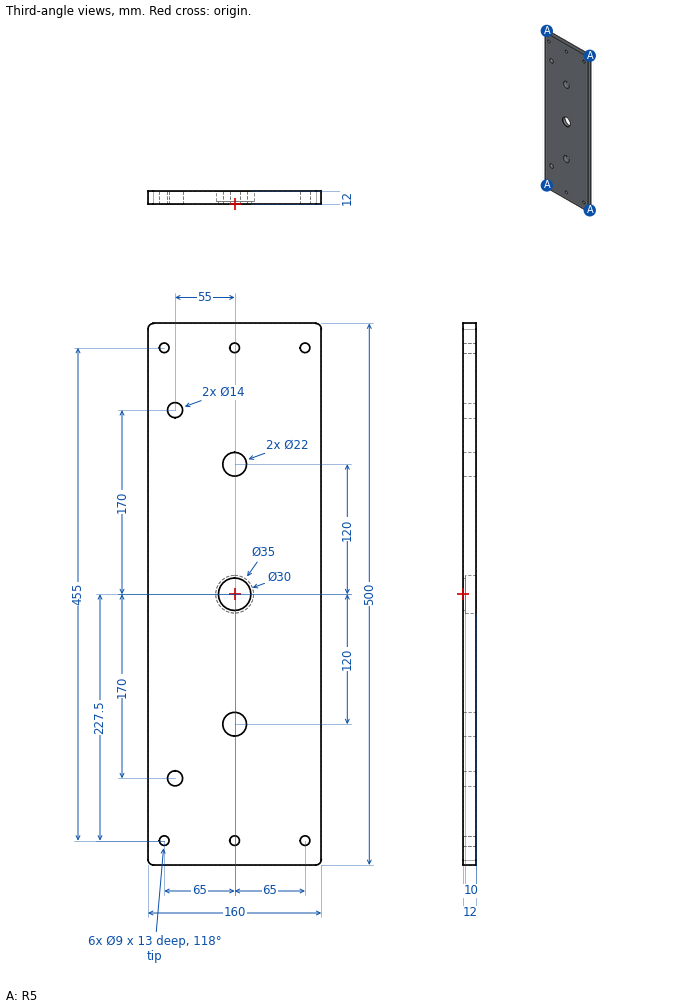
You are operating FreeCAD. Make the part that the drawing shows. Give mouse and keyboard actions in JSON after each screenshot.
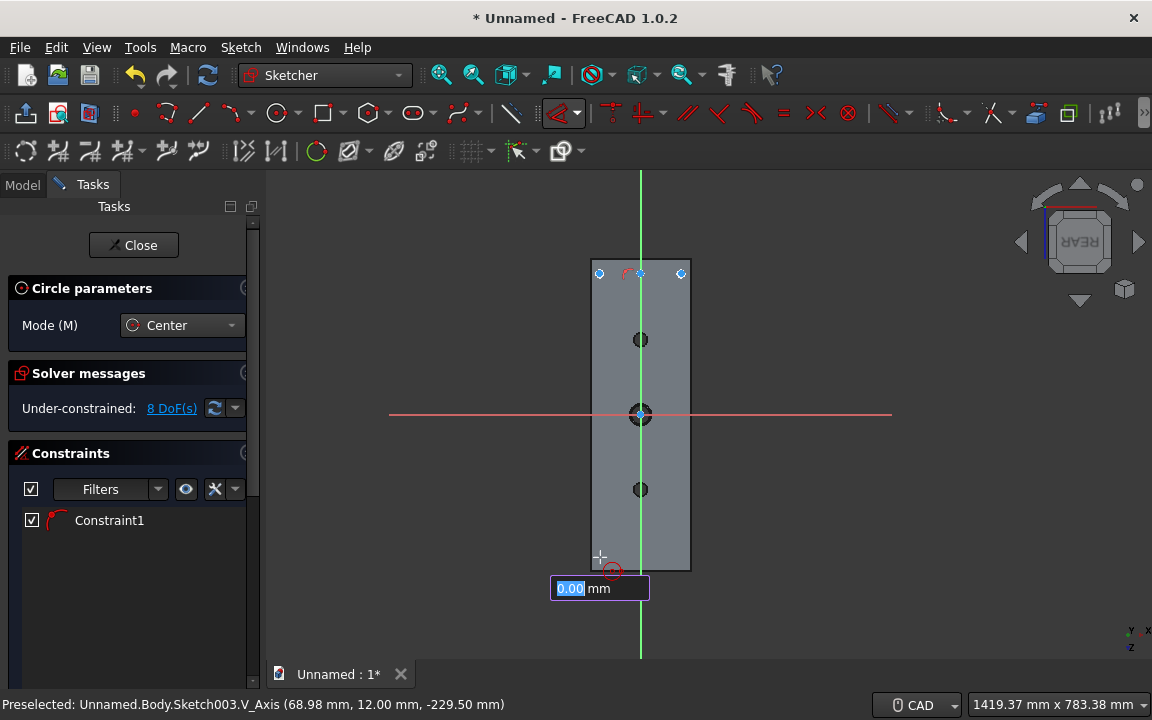
{"action": "scroll", "coordinate": [602, 555], "scroll_direction": "up", "scroll_amount": 9}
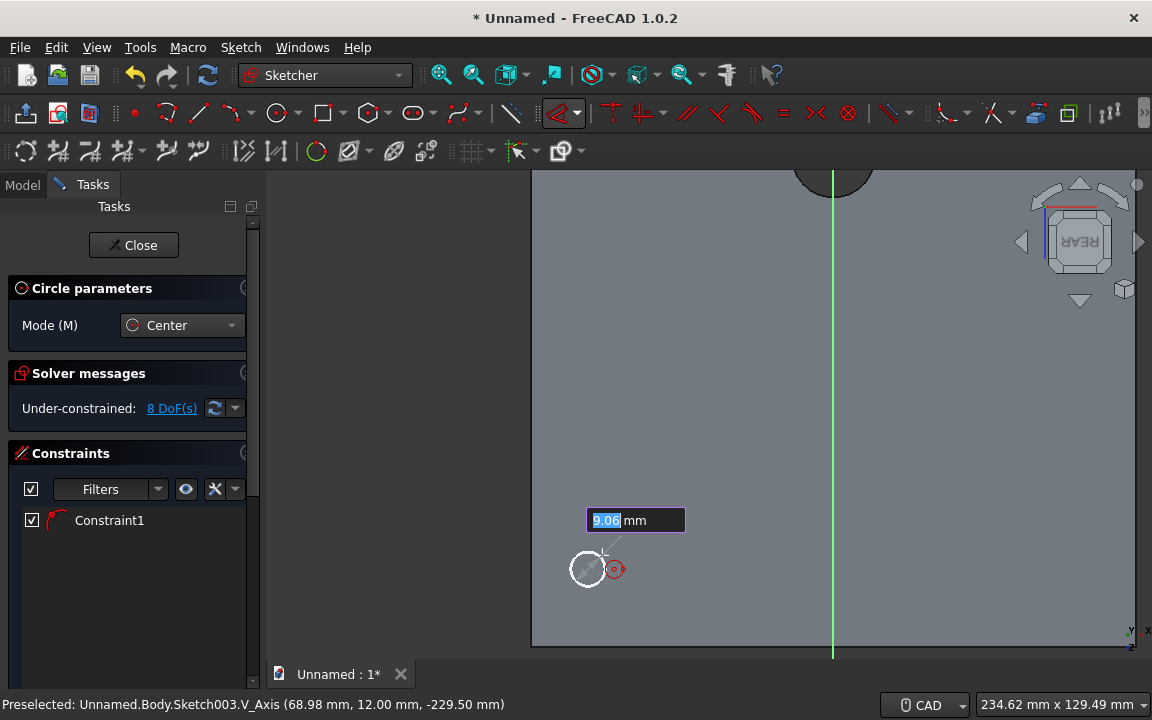
{"action": "left_click", "coordinate": [600, 550]}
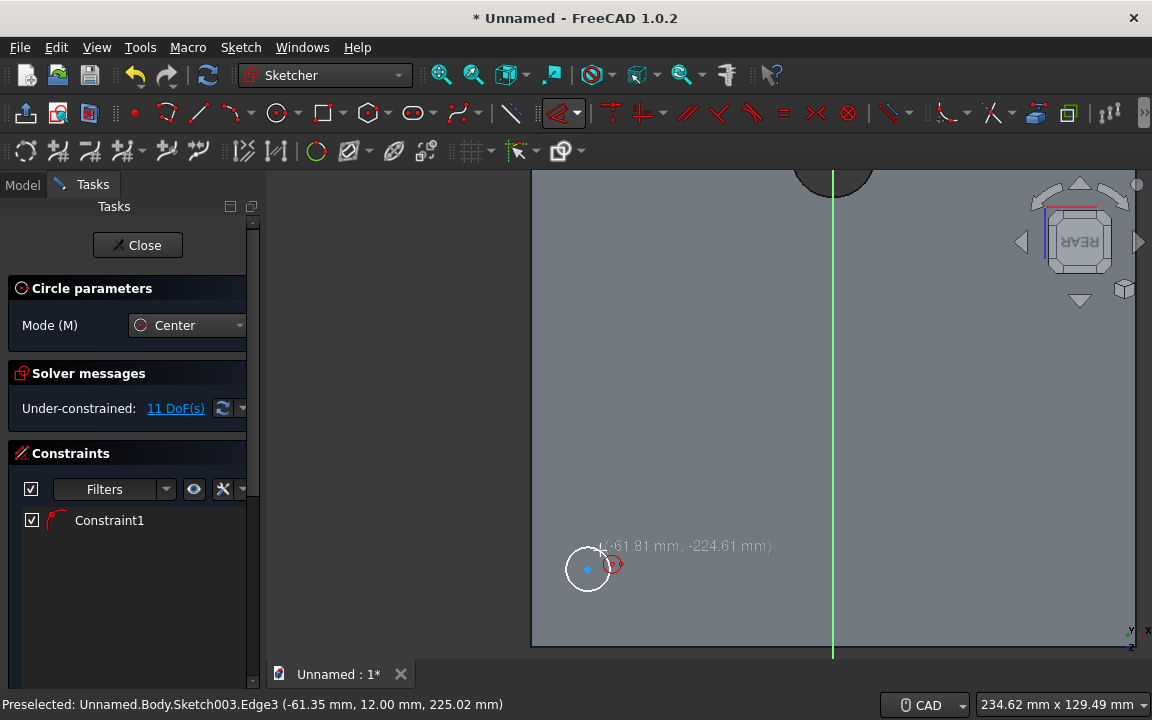
{"action": "scroll", "coordinate": [833, 562], "scroll_direction": "up", "scroll_amount": 2}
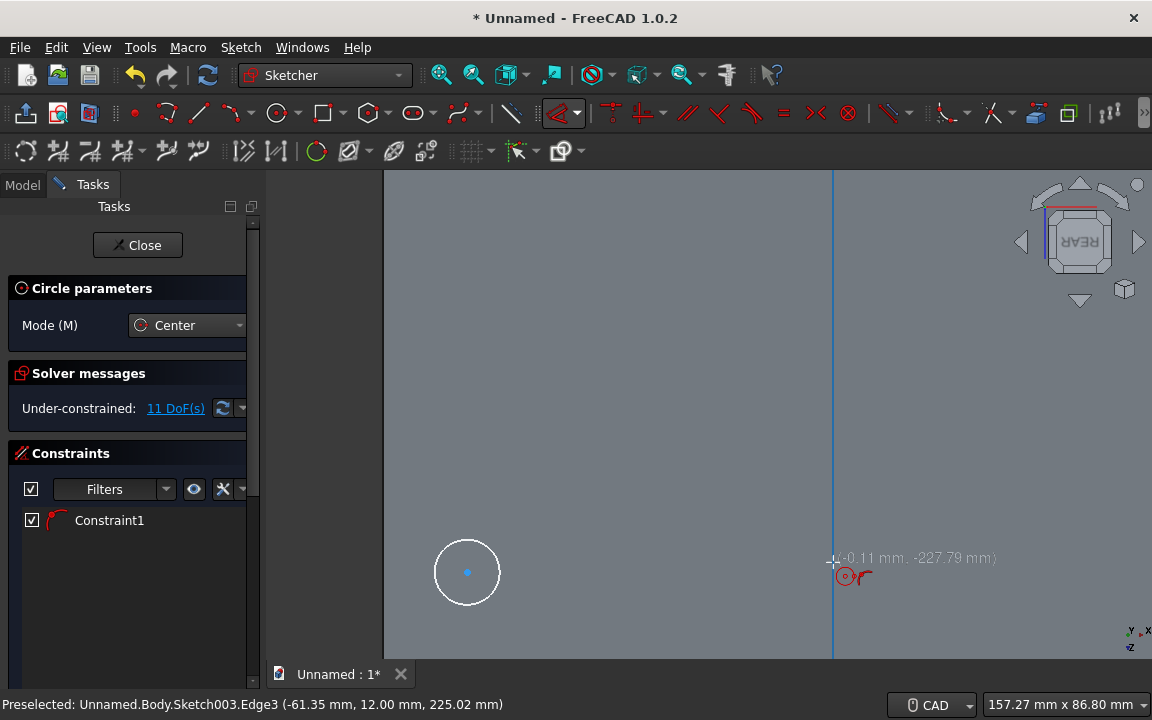
{"action": "scroll", "coordinate": [616, 556], "scroll_direction": "down", "scroll_amount": 11}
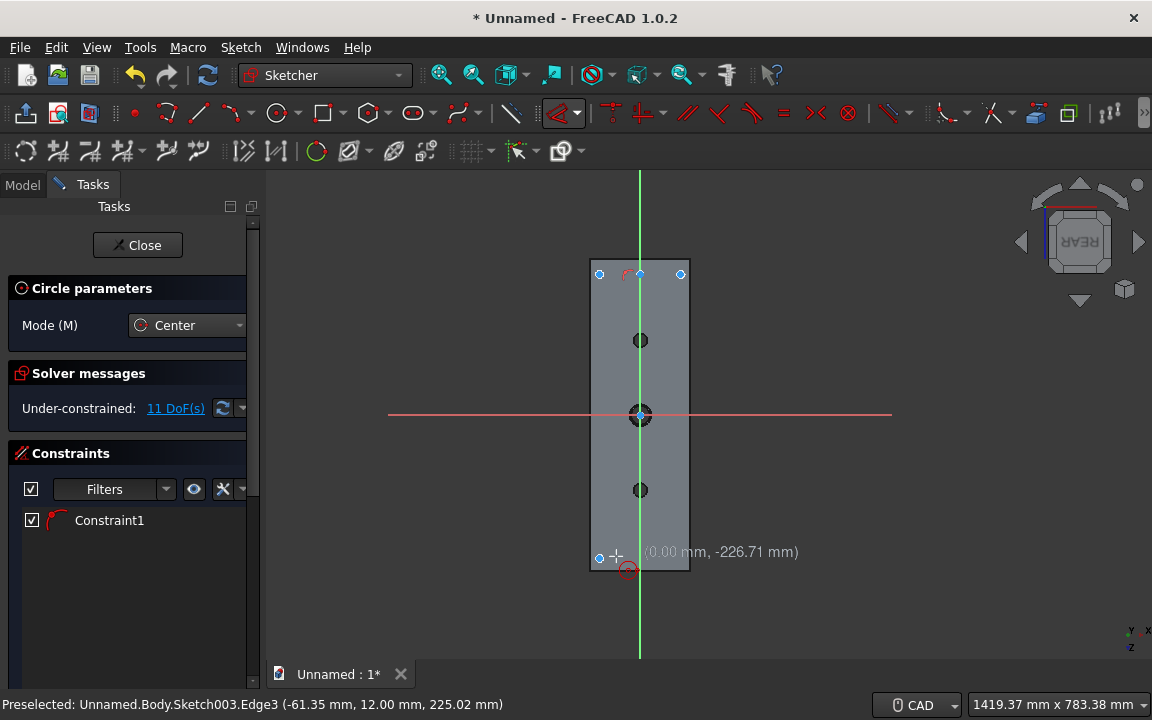
{"action": "left_click", "coordinate": [640, 557]}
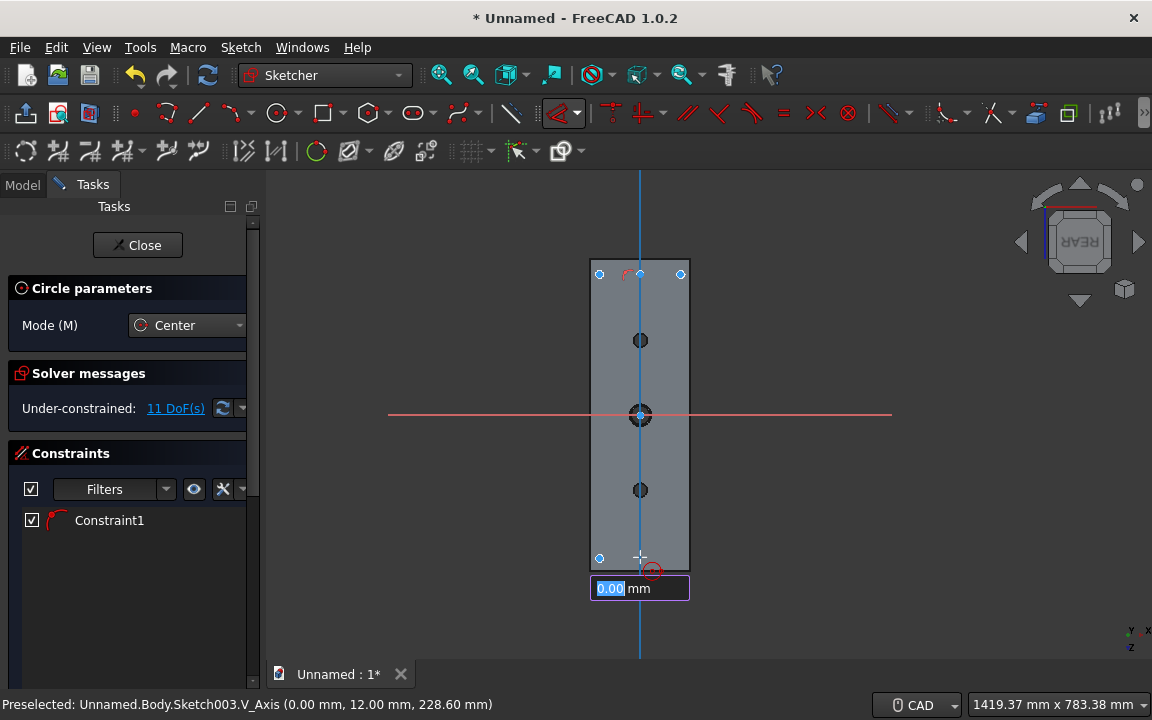
{"action": "scroll", "coordinate": [643, 556], "scroll_direction": "up", "scroll_amount": 9}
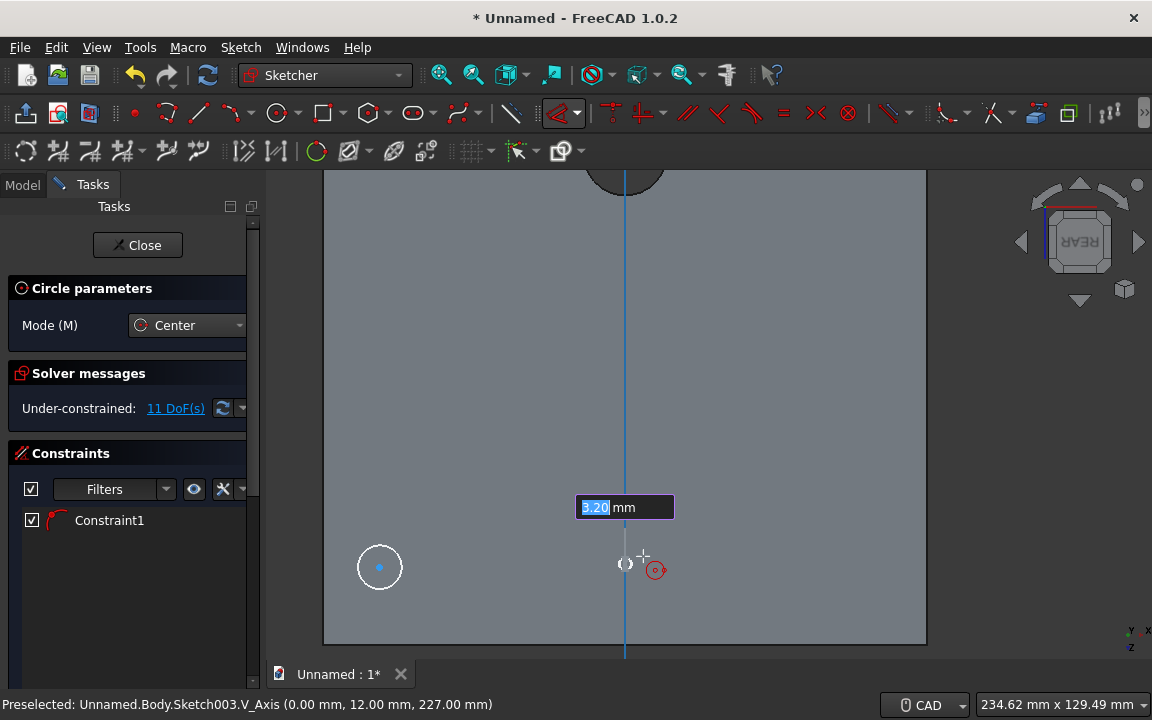
{"action": "left_click", "coordinate": [641, 554]}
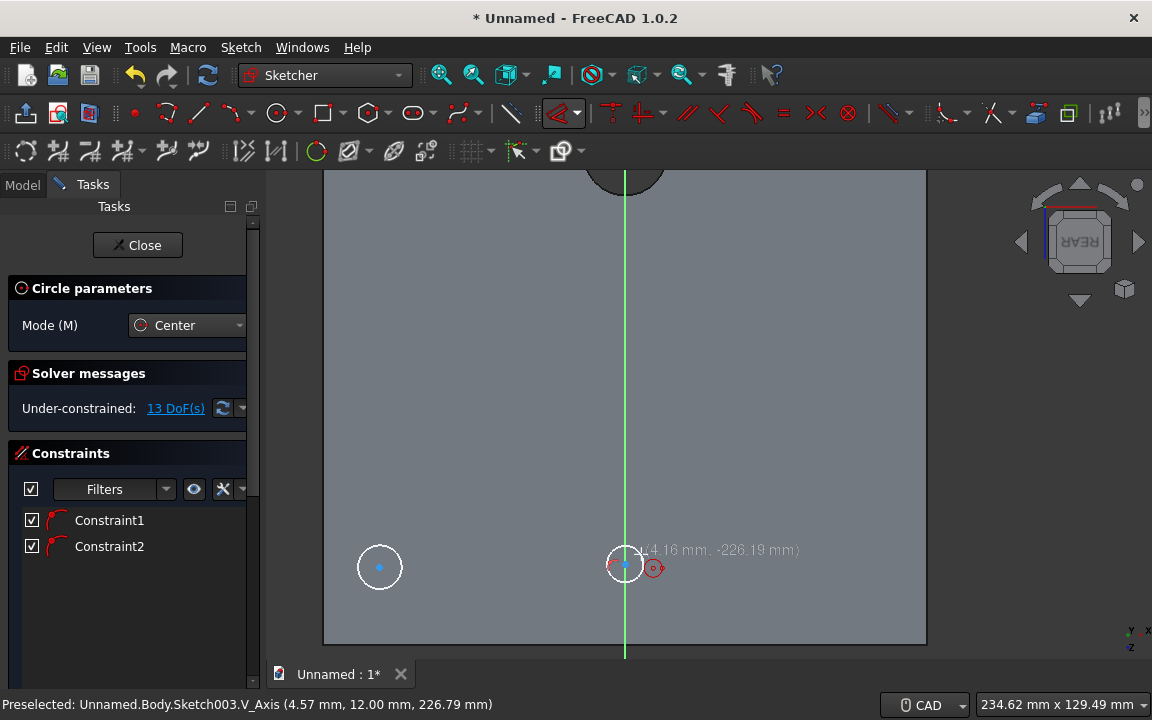
{"action": "scroll", "coordinate": [871, 560], "scroll_direction": "up", "scroll_amount": 2}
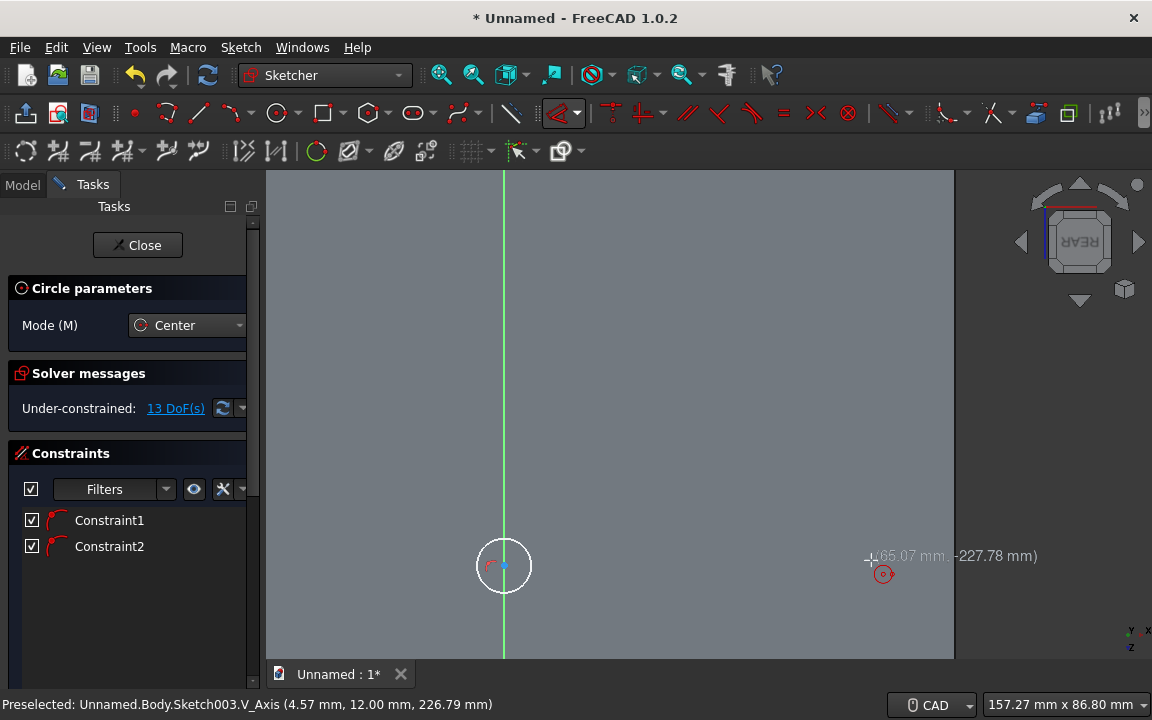
{"action": "scroll", "coordinate": [657, 556], "scroll_direction": "down", "scroll_amount": 11}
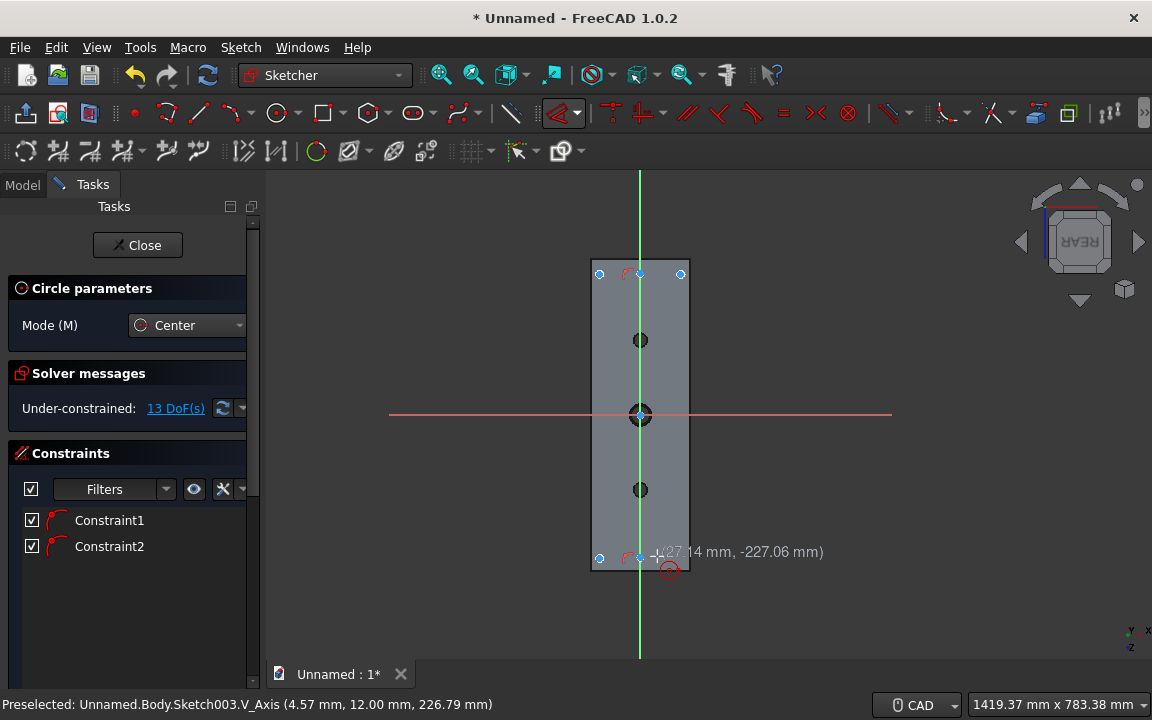
{"action": "left_click", "coordinate": [681, 557]}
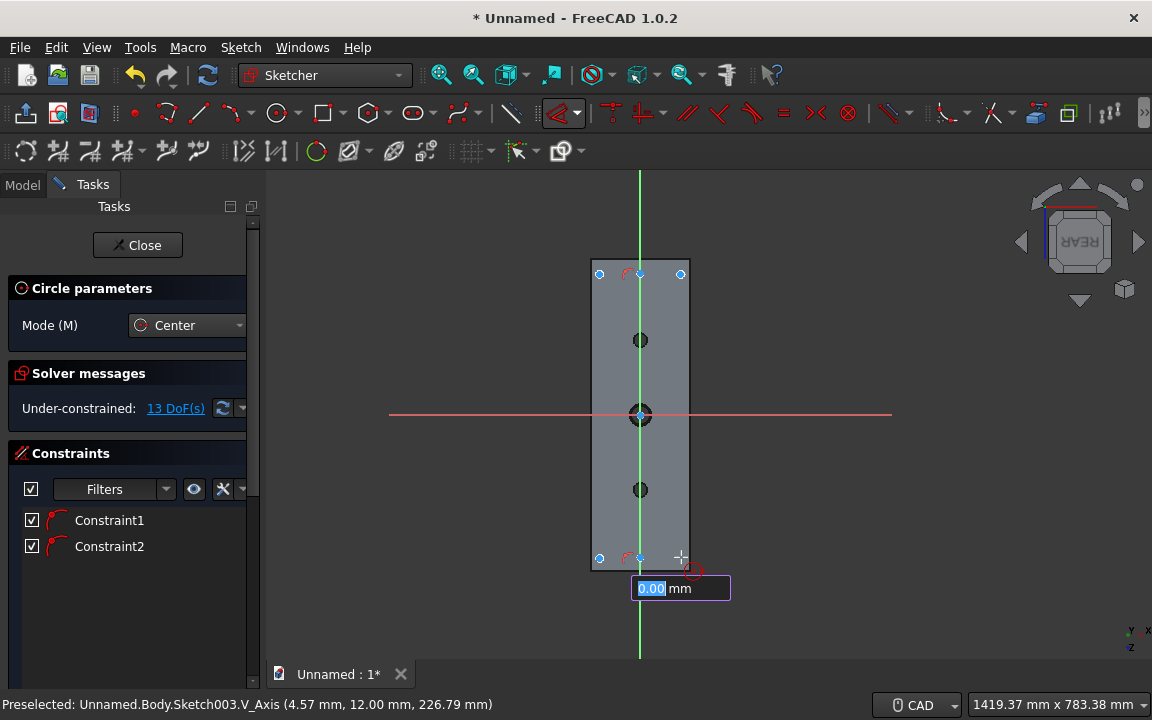
{"action": "scroll", "coordinate": [683, 555], "scroll_direction": "up", "scroll_amount": 9}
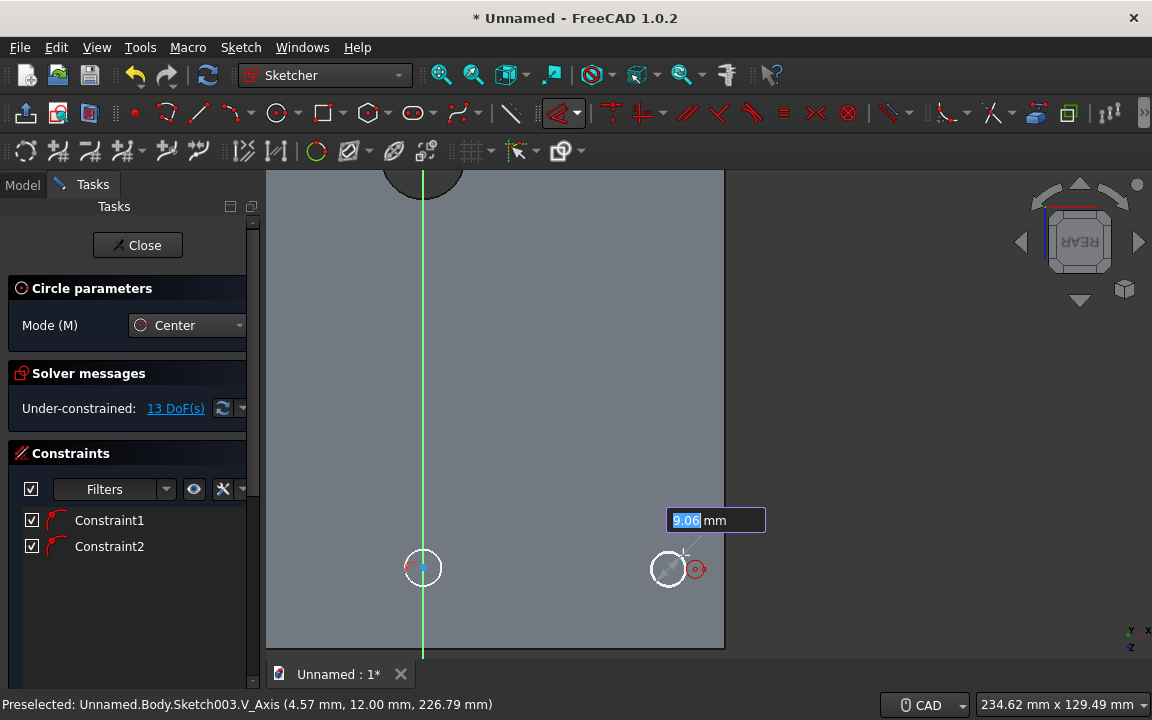
{"action": "left_click", "coordinate": [681, 552]}
{"action": "key", "text": "Escape"}